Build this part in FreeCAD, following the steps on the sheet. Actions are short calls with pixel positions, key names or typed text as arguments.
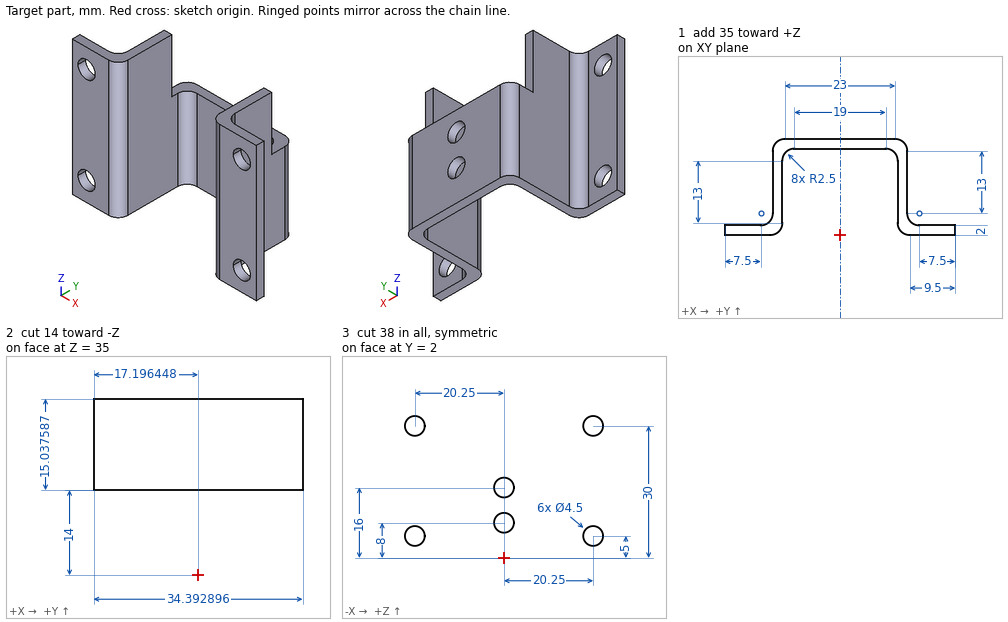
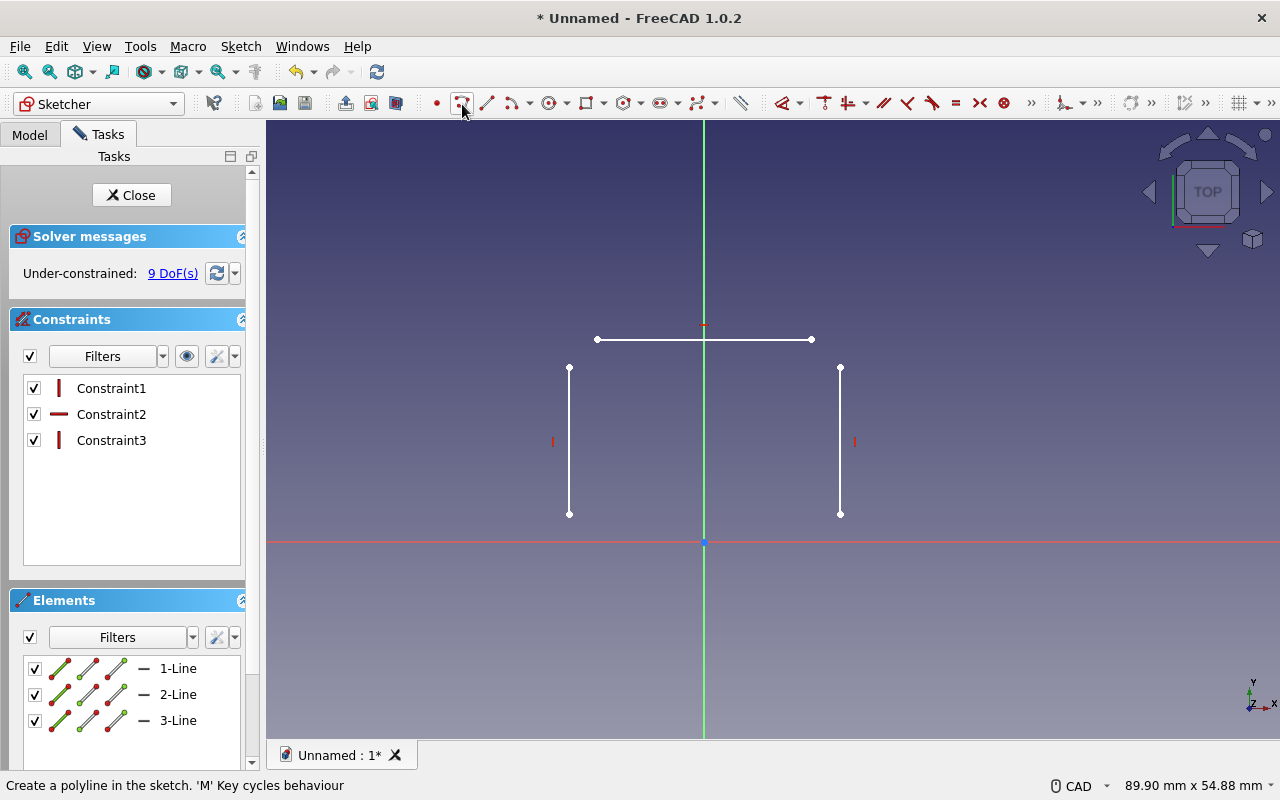
click(868, 542)
click(975, 533)
click(975, 520)
click(890, 520)
right_click(890, 520)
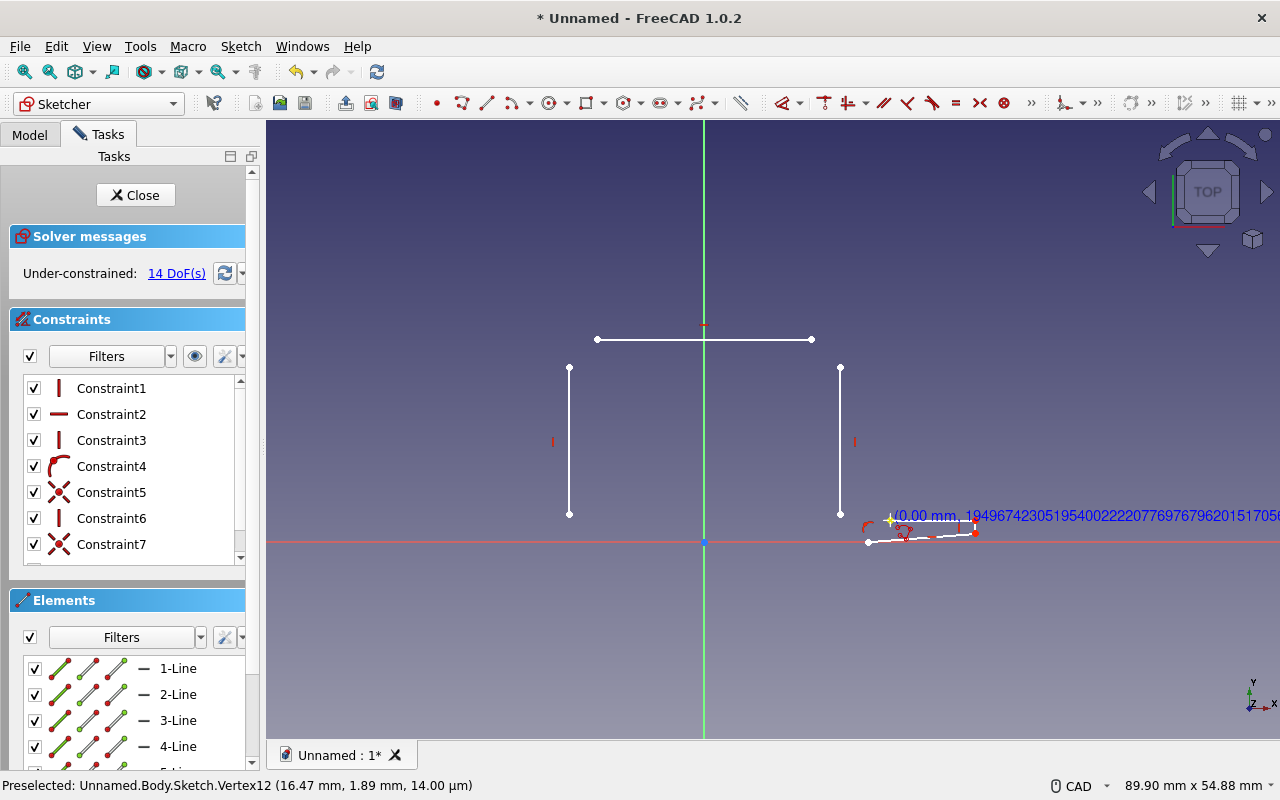
key(g)
key(l)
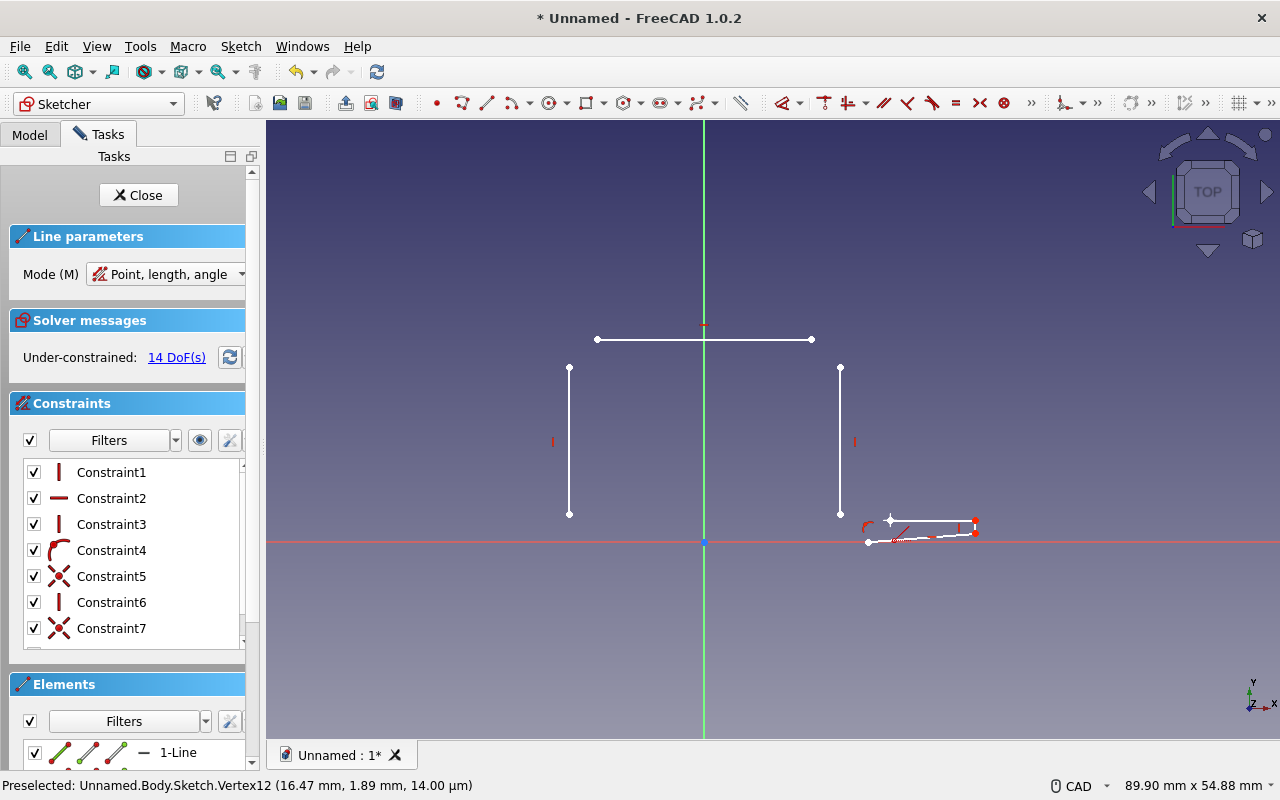
click(862, 492)
click(862, 345)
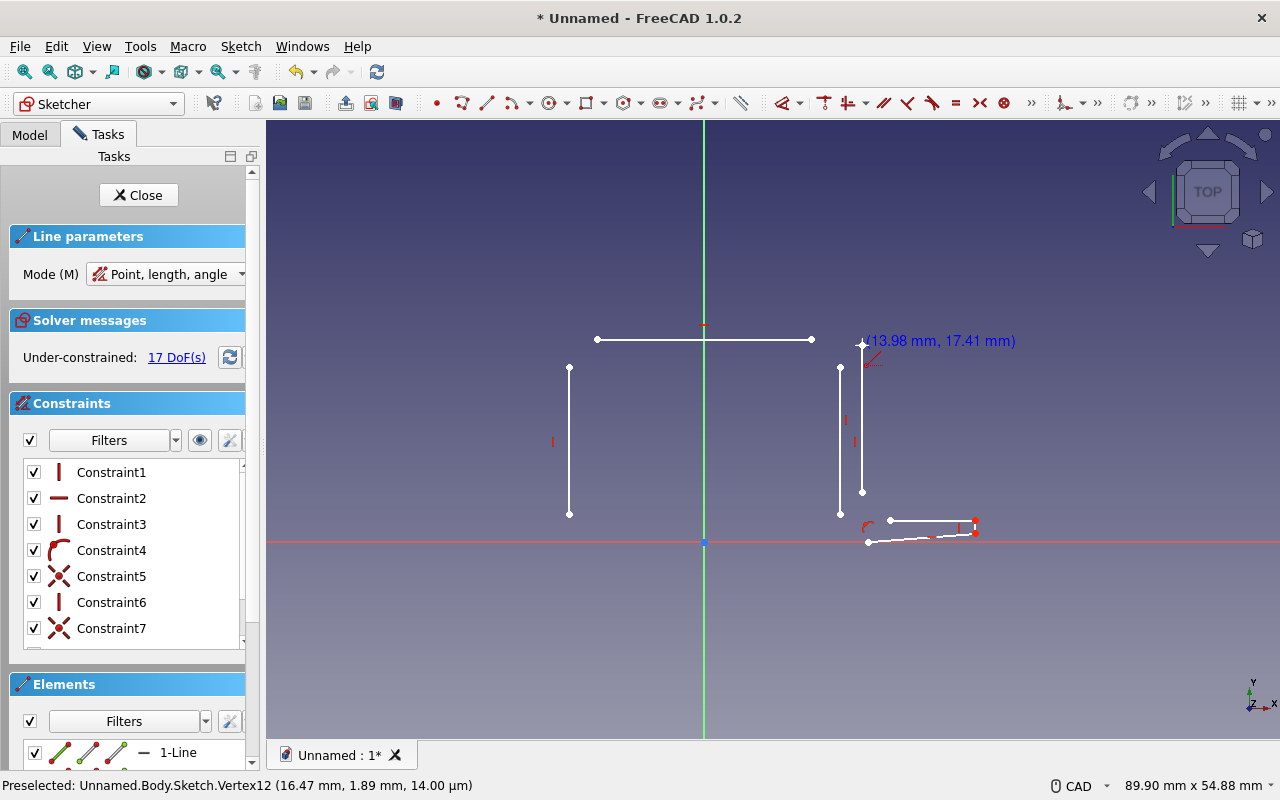
click(834, 317)
click(575, 317)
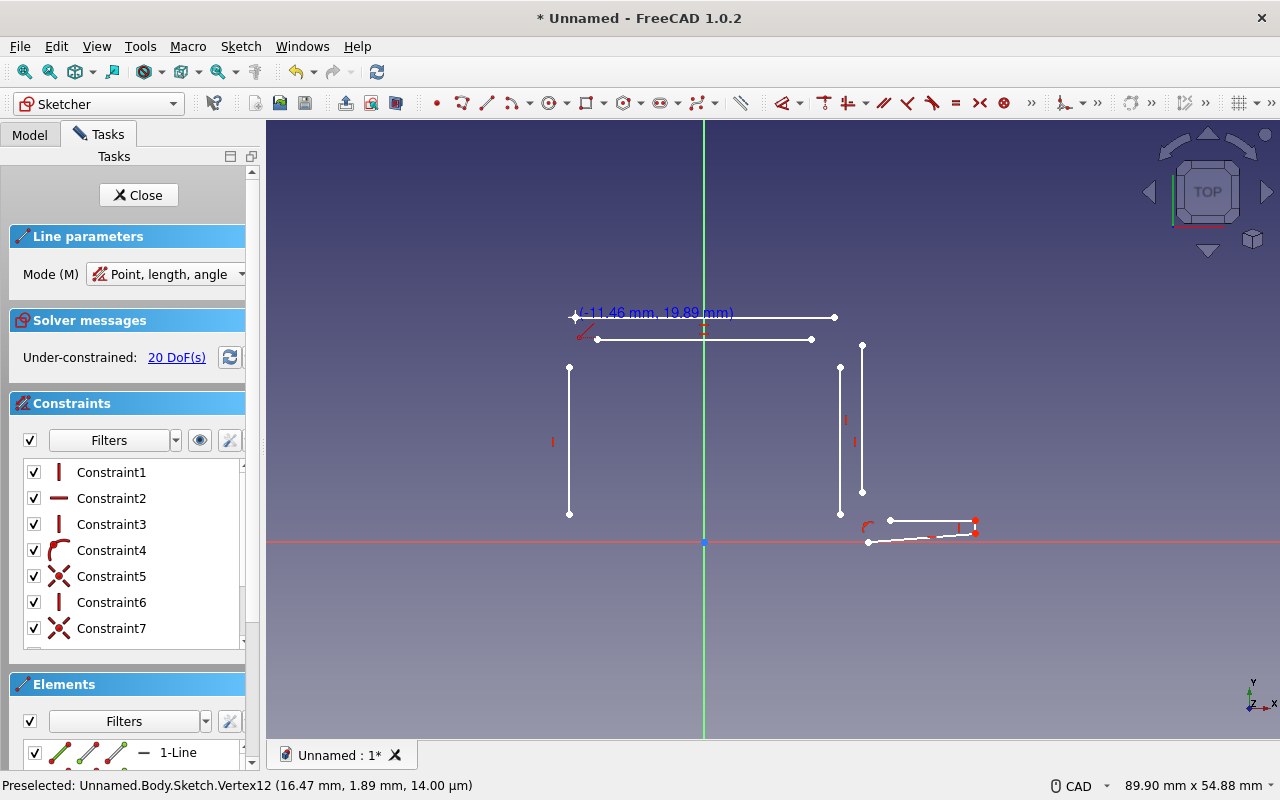
click(546, 345)
click(546, 492)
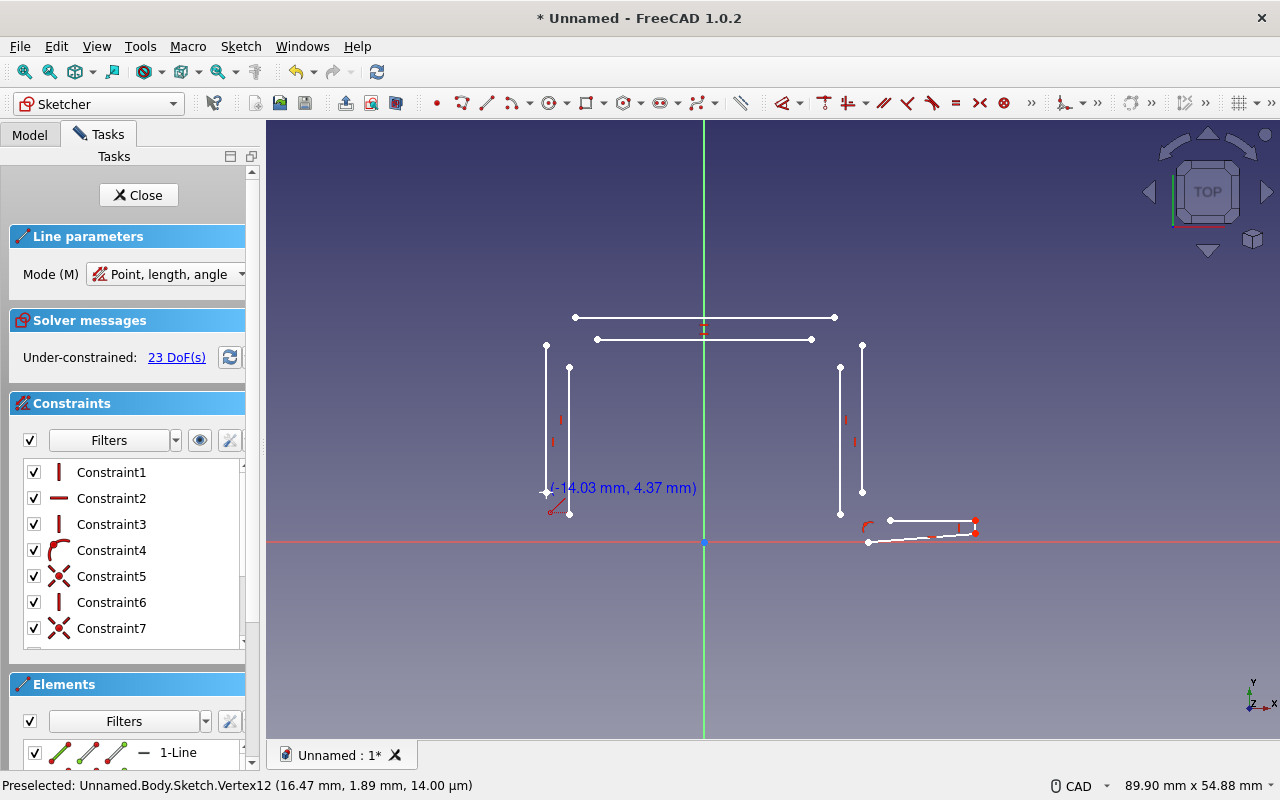
click(462, 104)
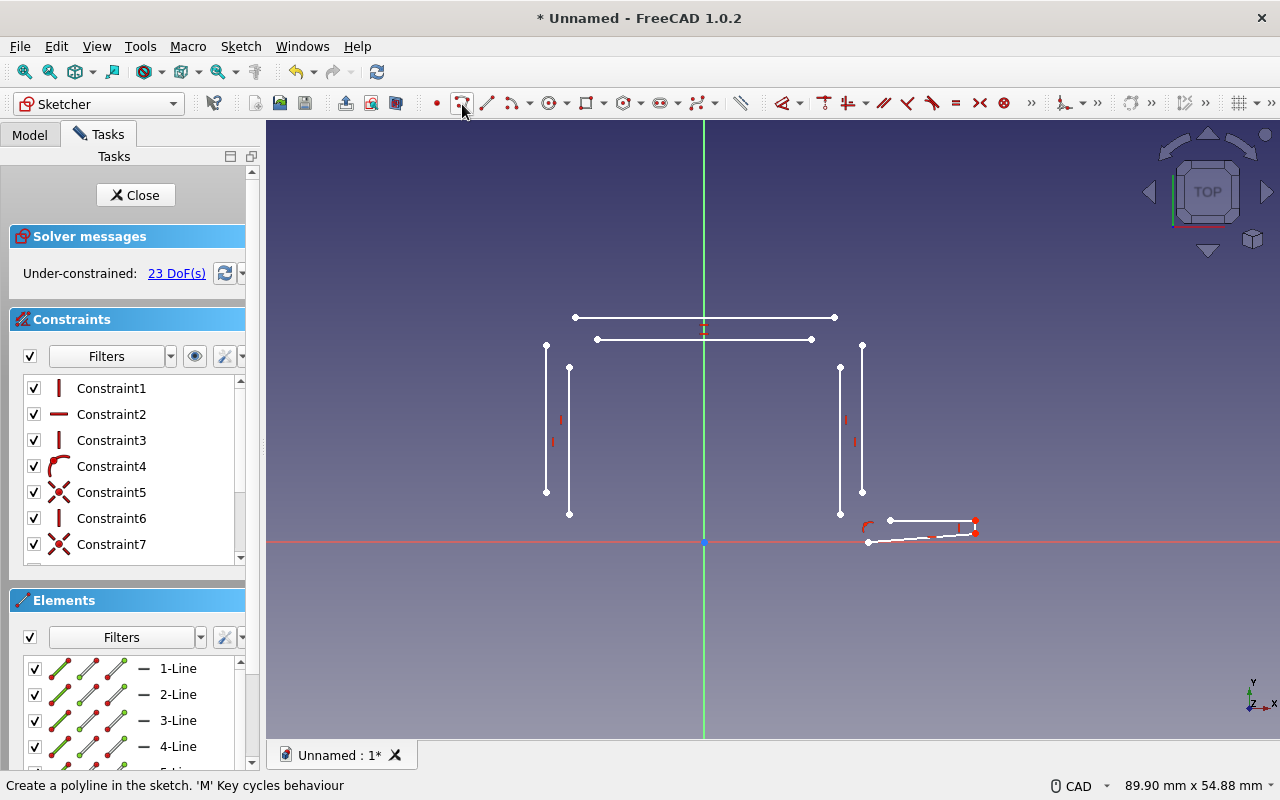
click(518, 520)
click(434, 520)
click(434, 542)
click(541, 533)
right_click(541, 533)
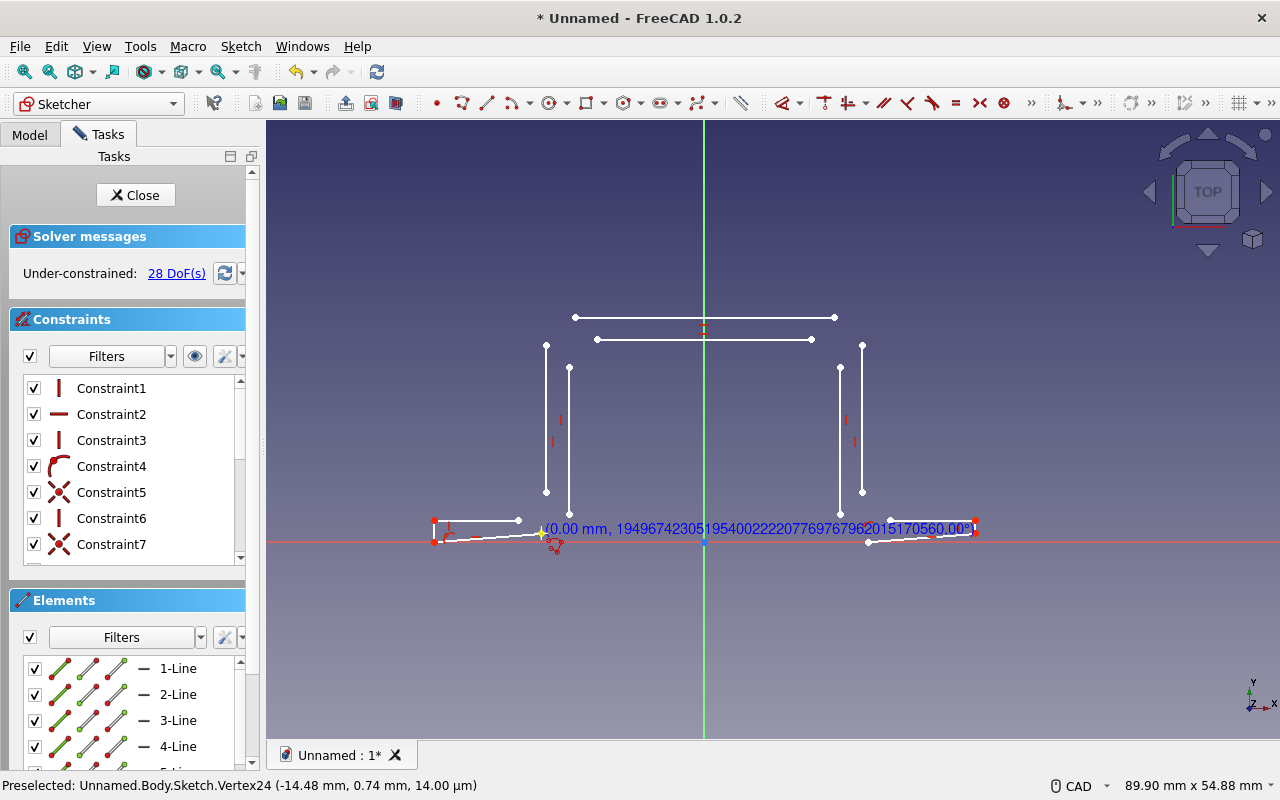
click(530, 104)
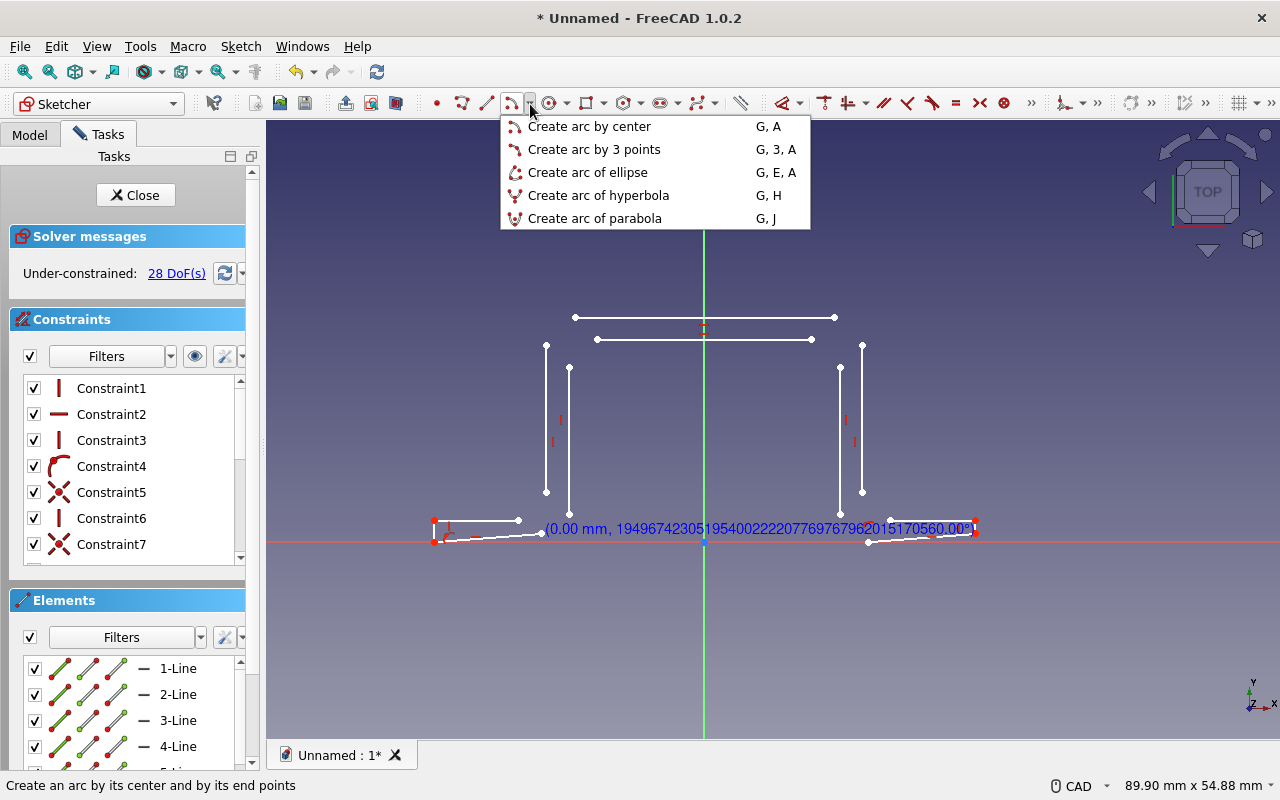
click(656, 150)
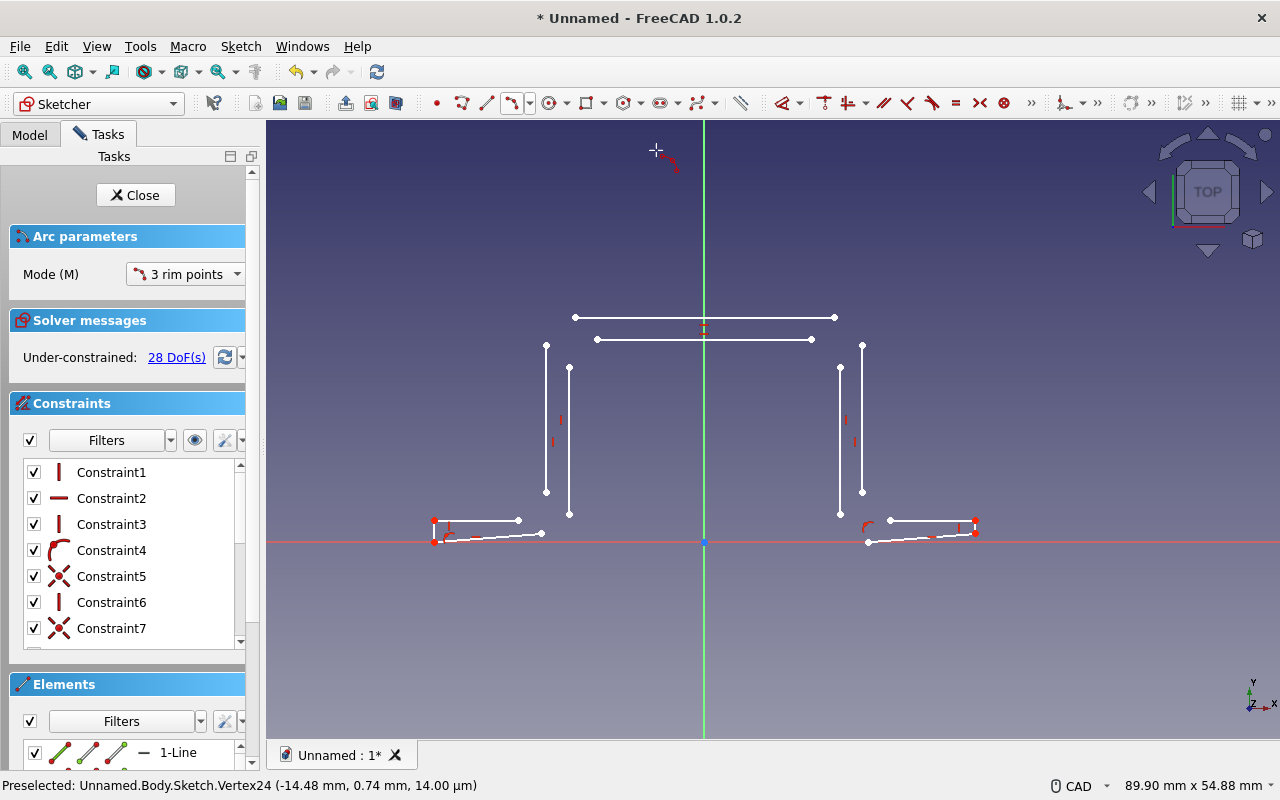
click(569, 368)
click(597, 340)